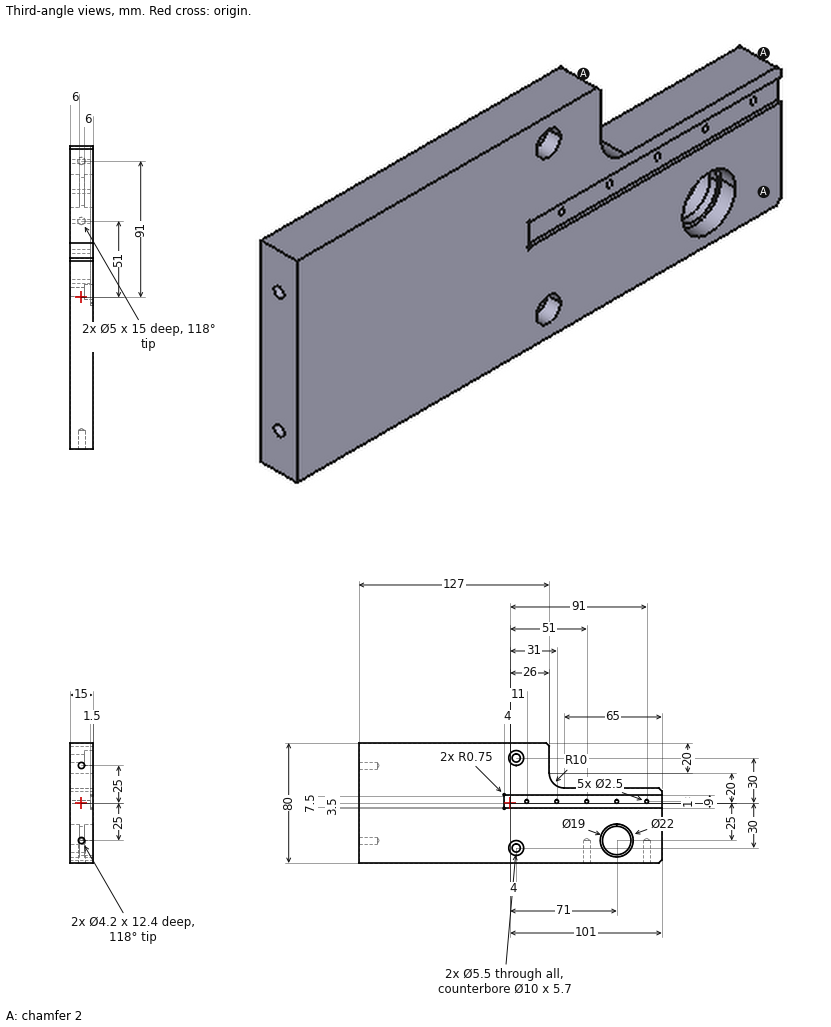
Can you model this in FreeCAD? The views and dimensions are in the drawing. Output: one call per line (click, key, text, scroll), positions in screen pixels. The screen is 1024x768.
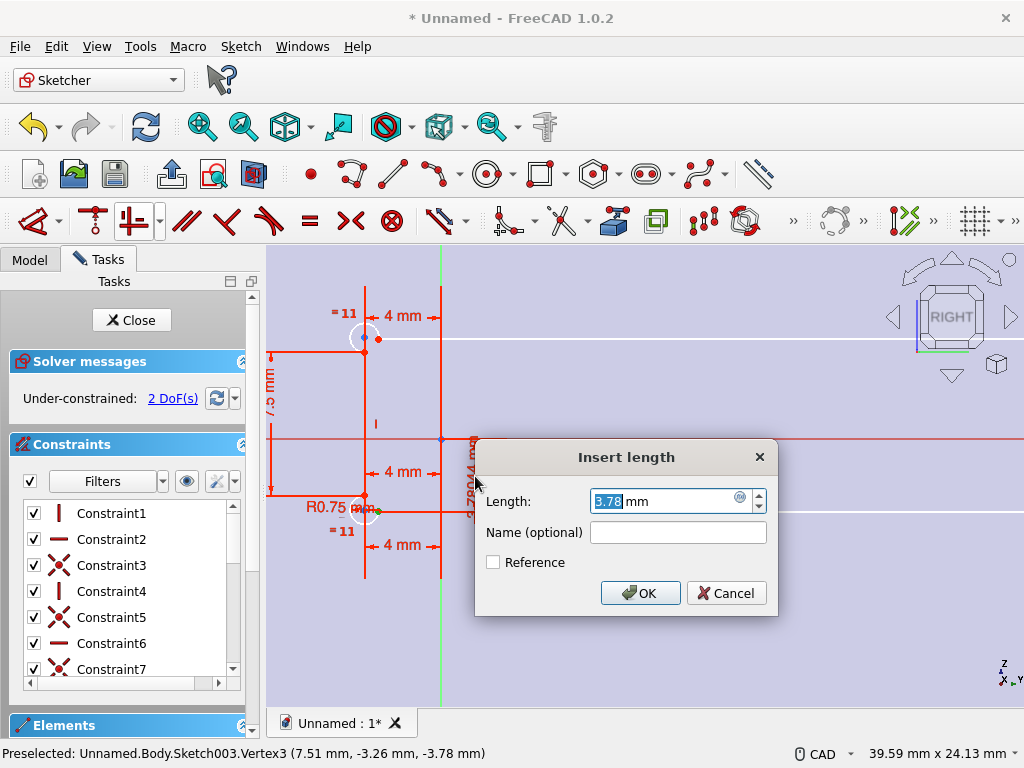
text(3.5)
key(Return)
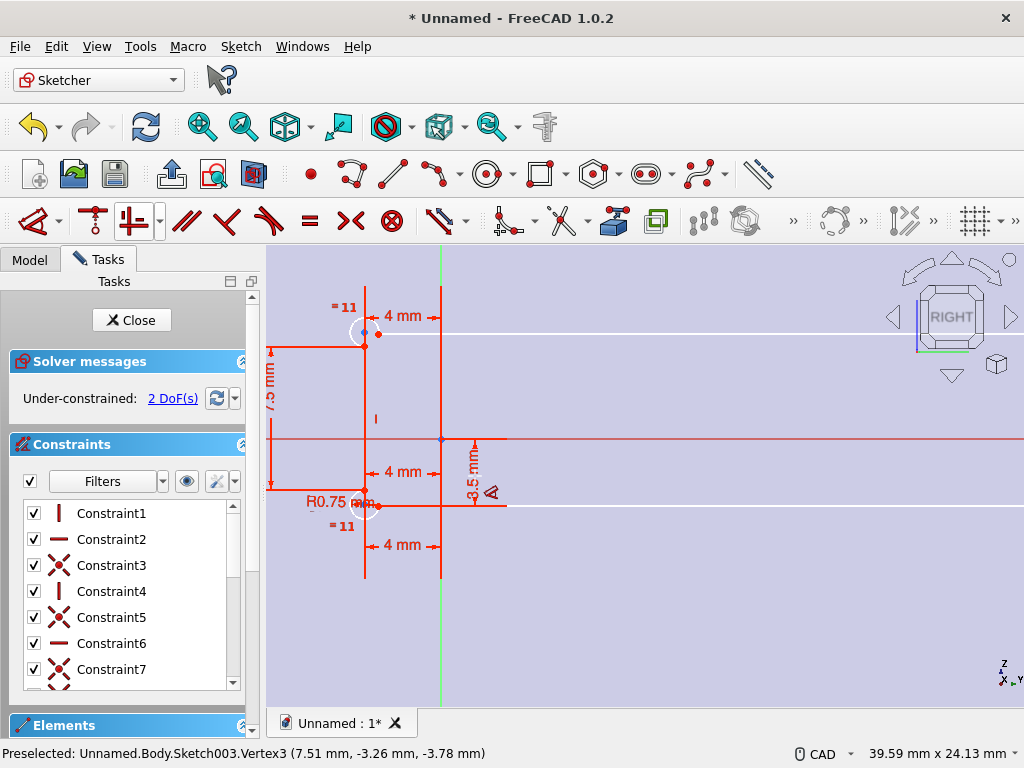
scroll(377, 490, down, 8)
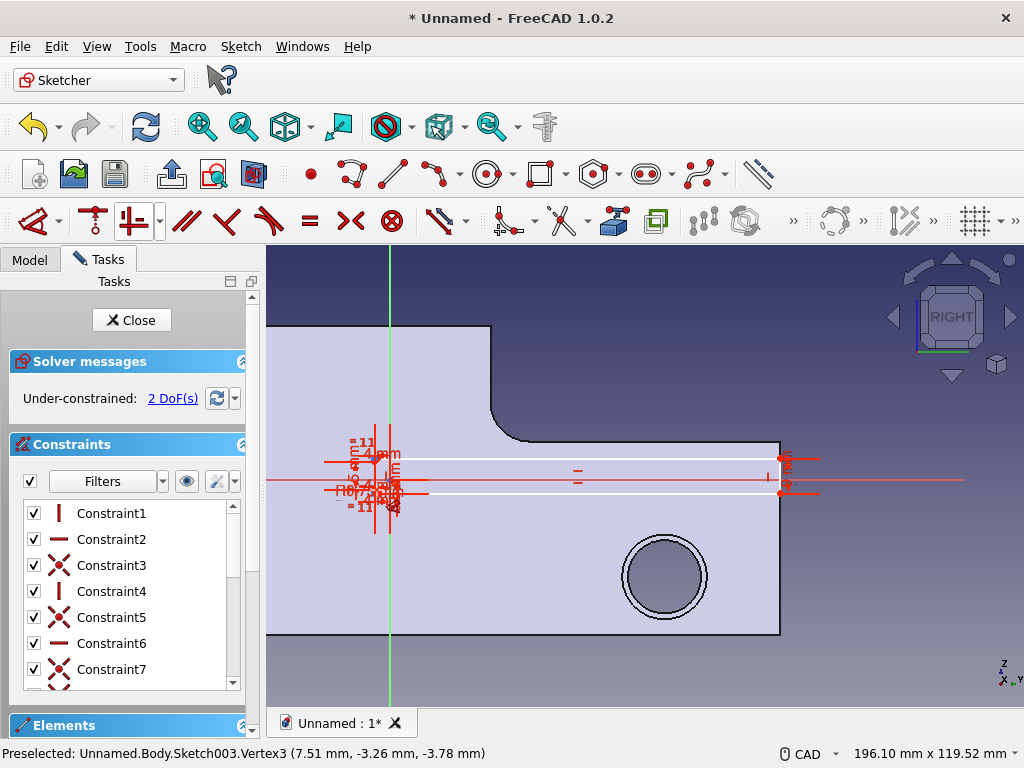
click(780, 494)
click(585, 528)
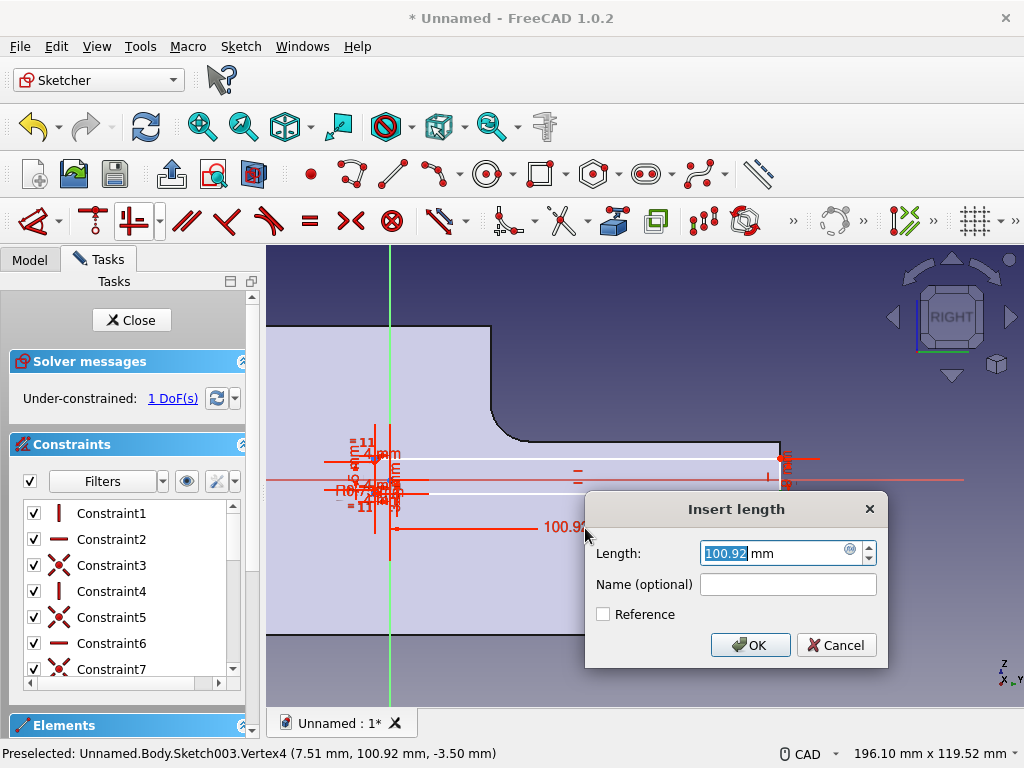
text(101)
key(Return)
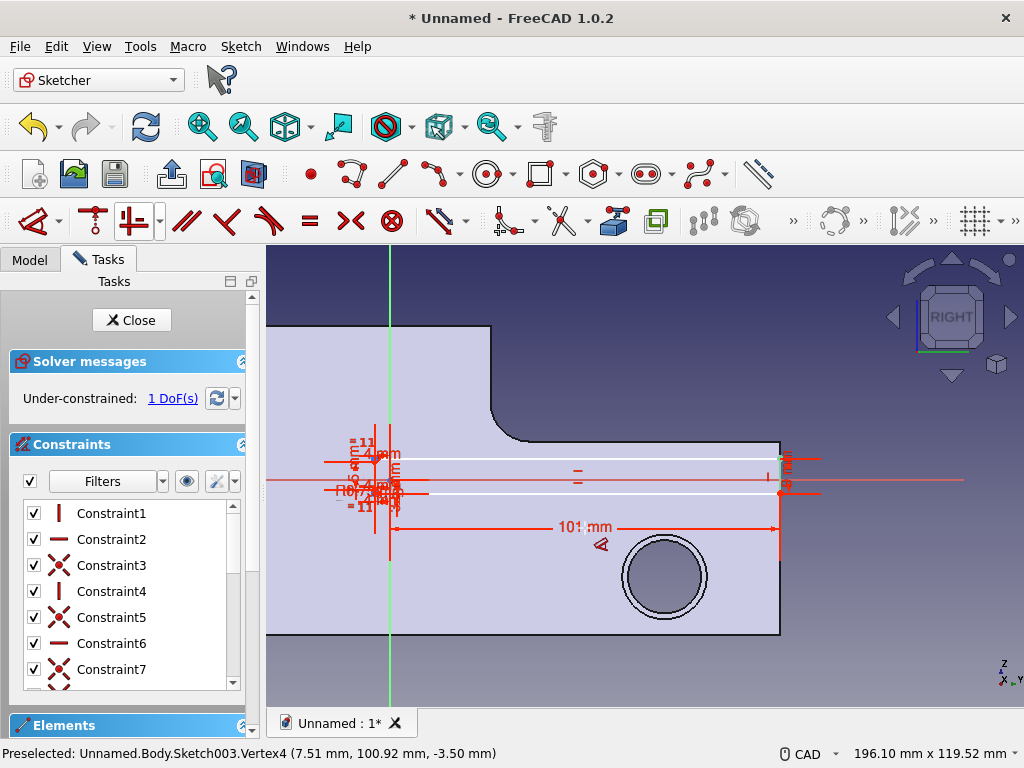
scroll(375, 493, up, 8)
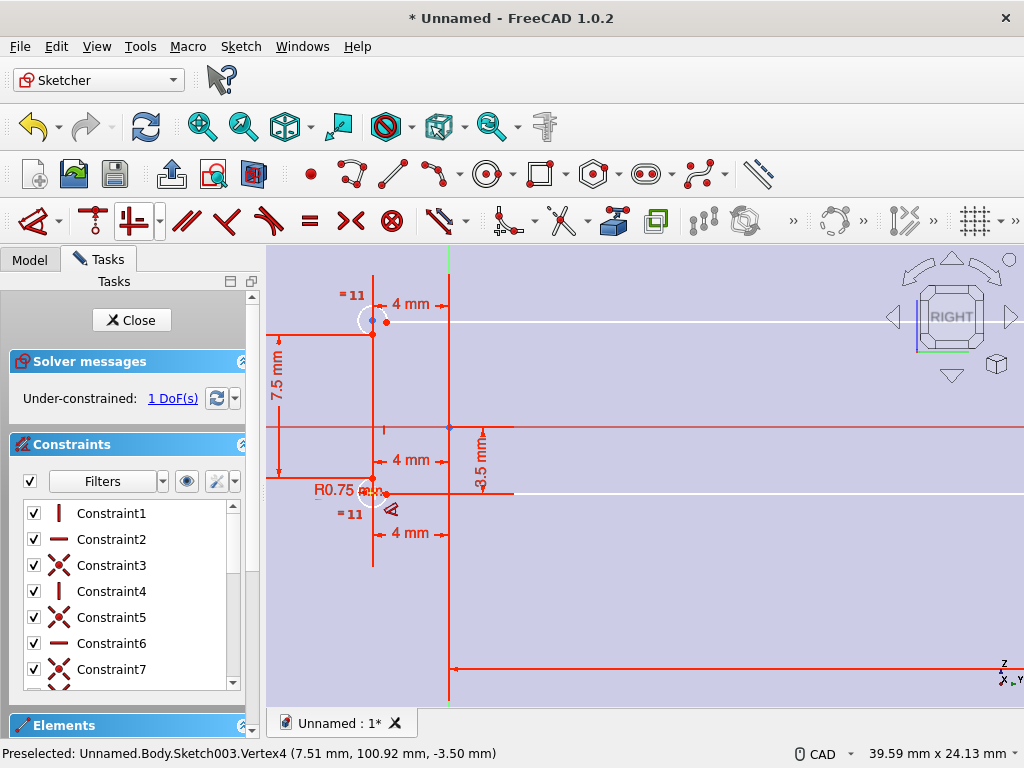
click(373, 493)
click(339, 460)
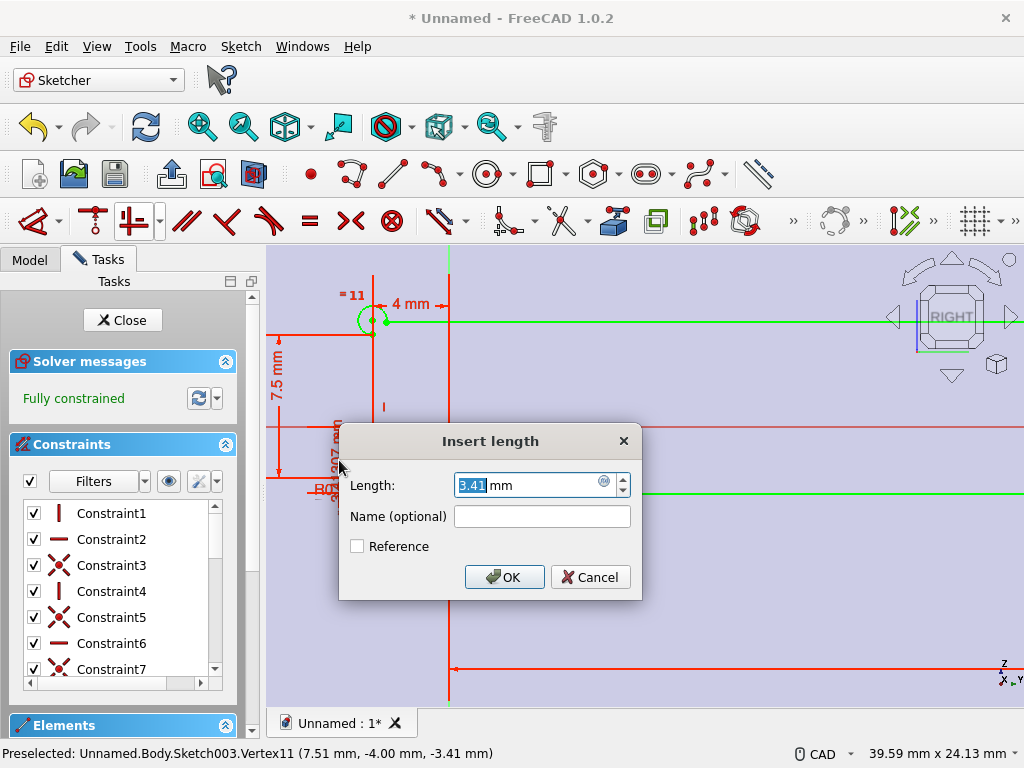
text(3.5)
key(Return)
key(Escape)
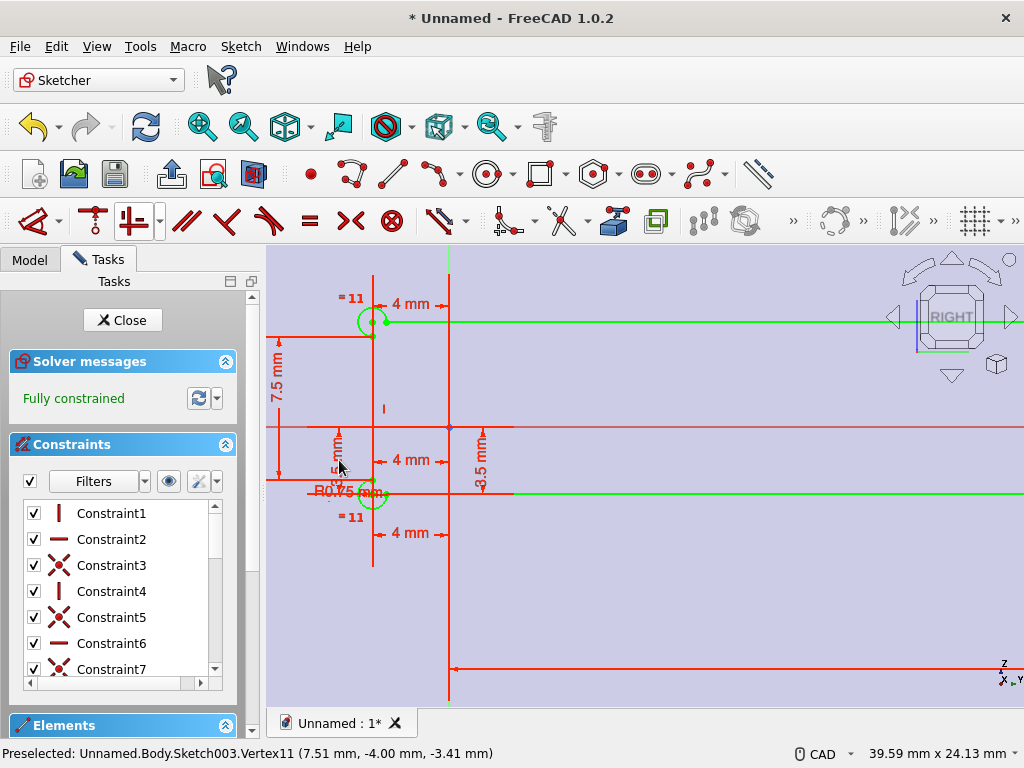
click(123, 320)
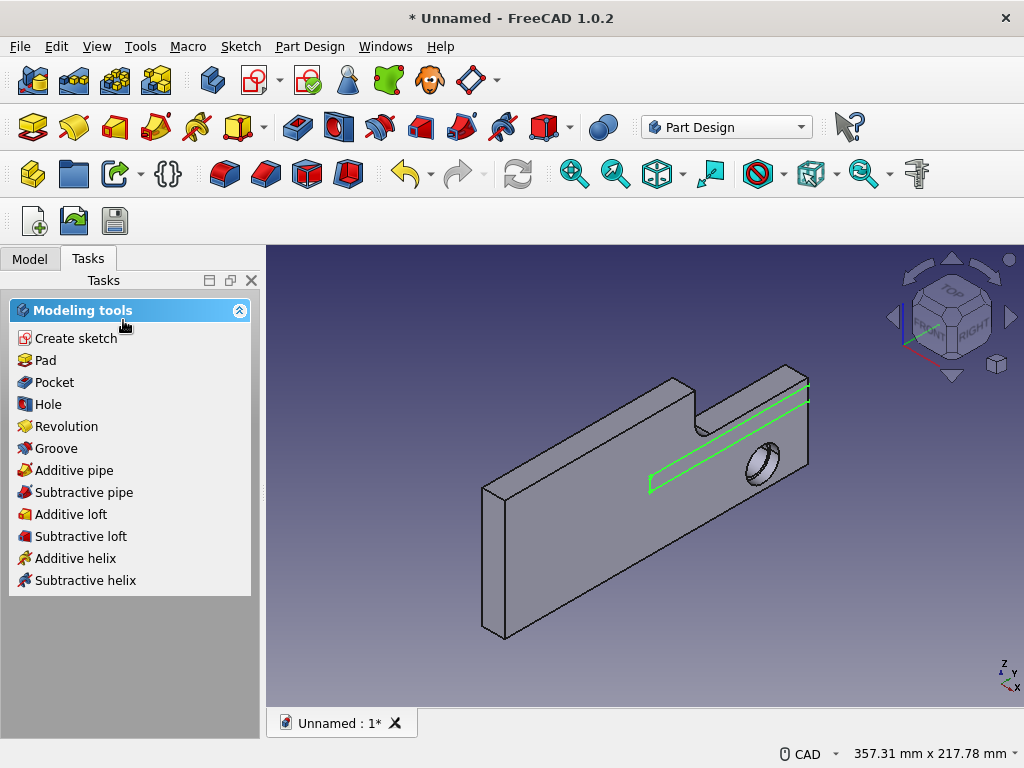
click(298, 128)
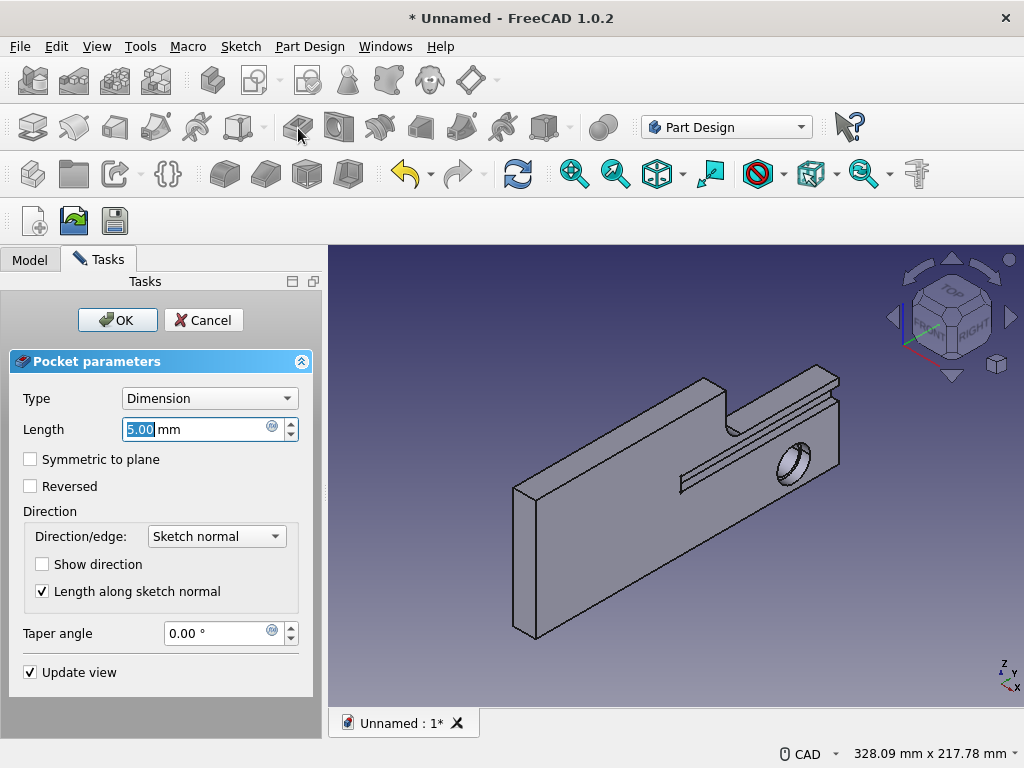
text(1.5)
key(Tab)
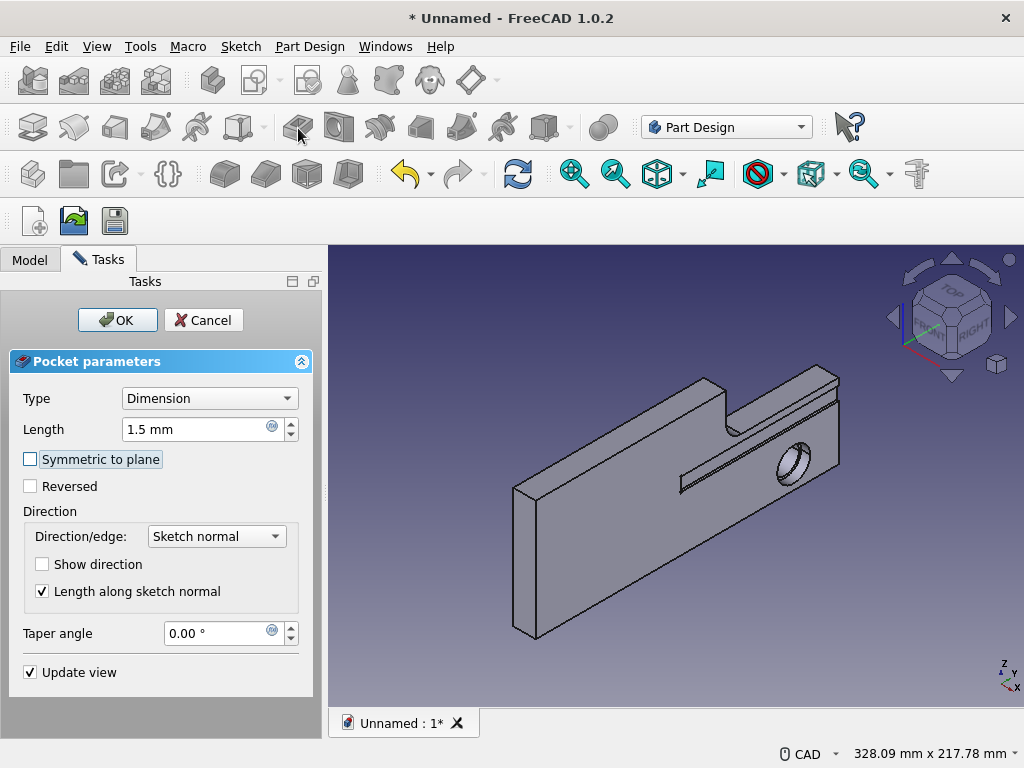
click(118, 320)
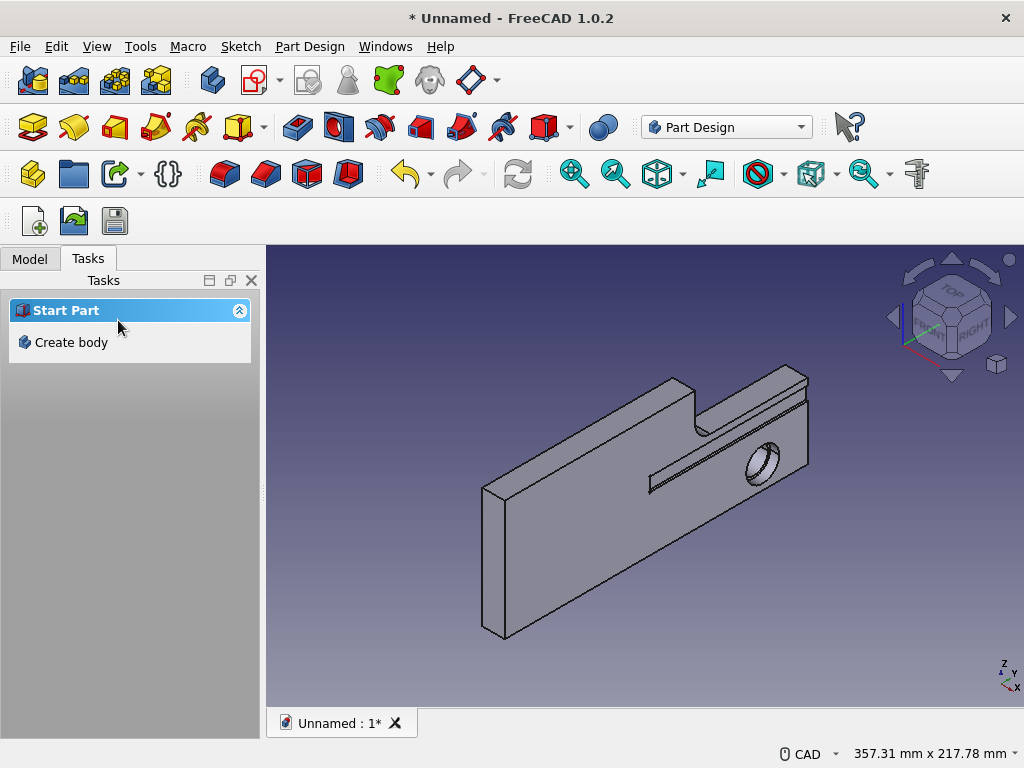
click(493, 582)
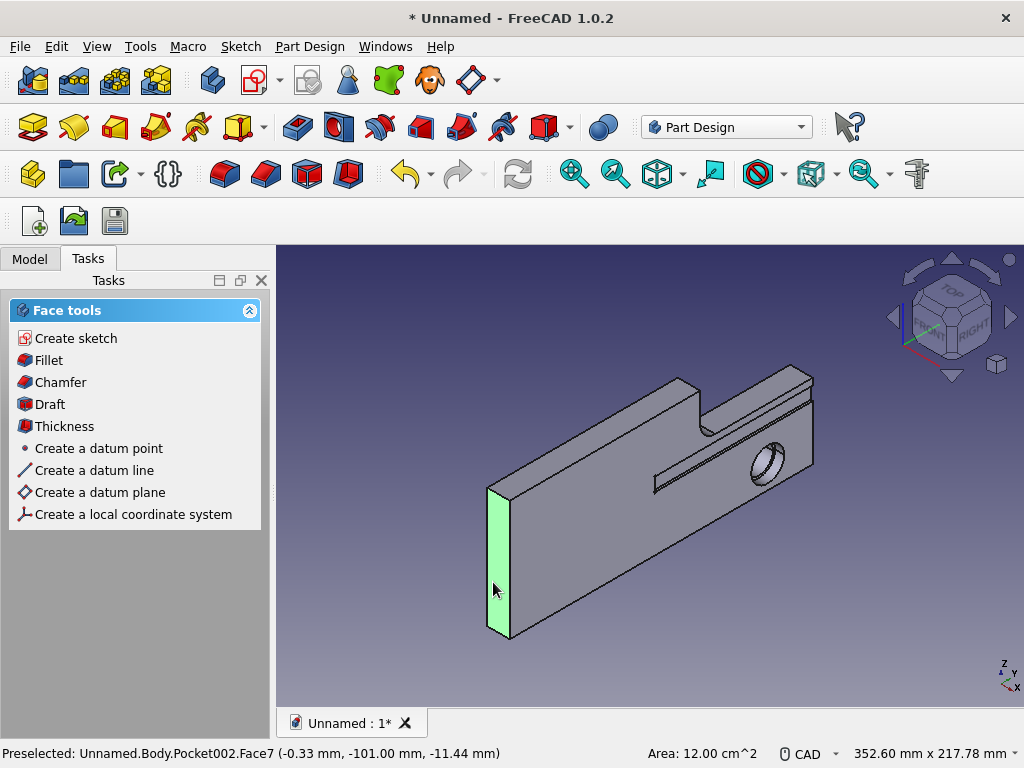
click(254, 80)